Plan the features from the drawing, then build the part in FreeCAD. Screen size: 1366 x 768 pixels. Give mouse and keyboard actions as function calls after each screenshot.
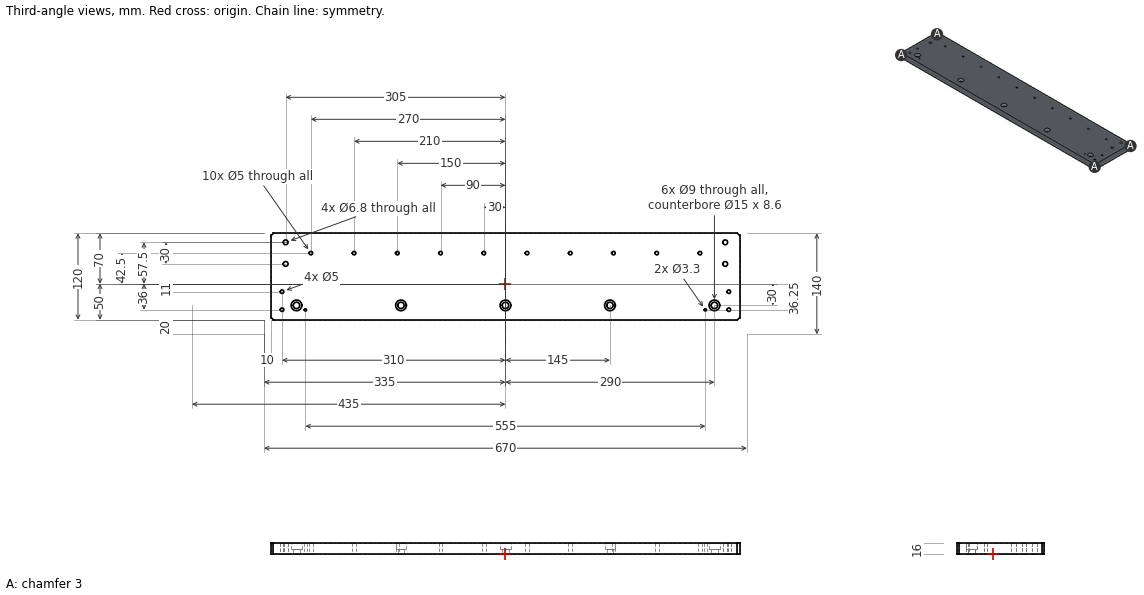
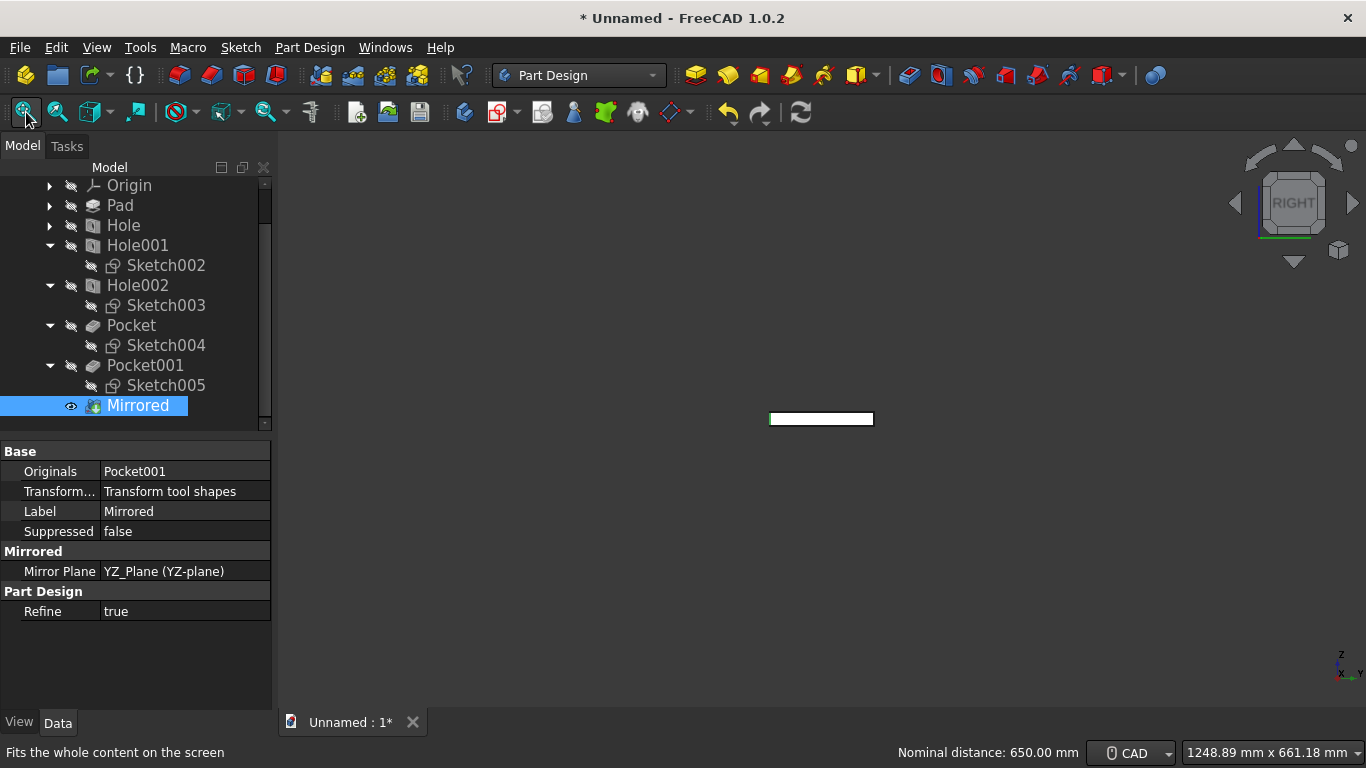
click(874, 418, ctrl)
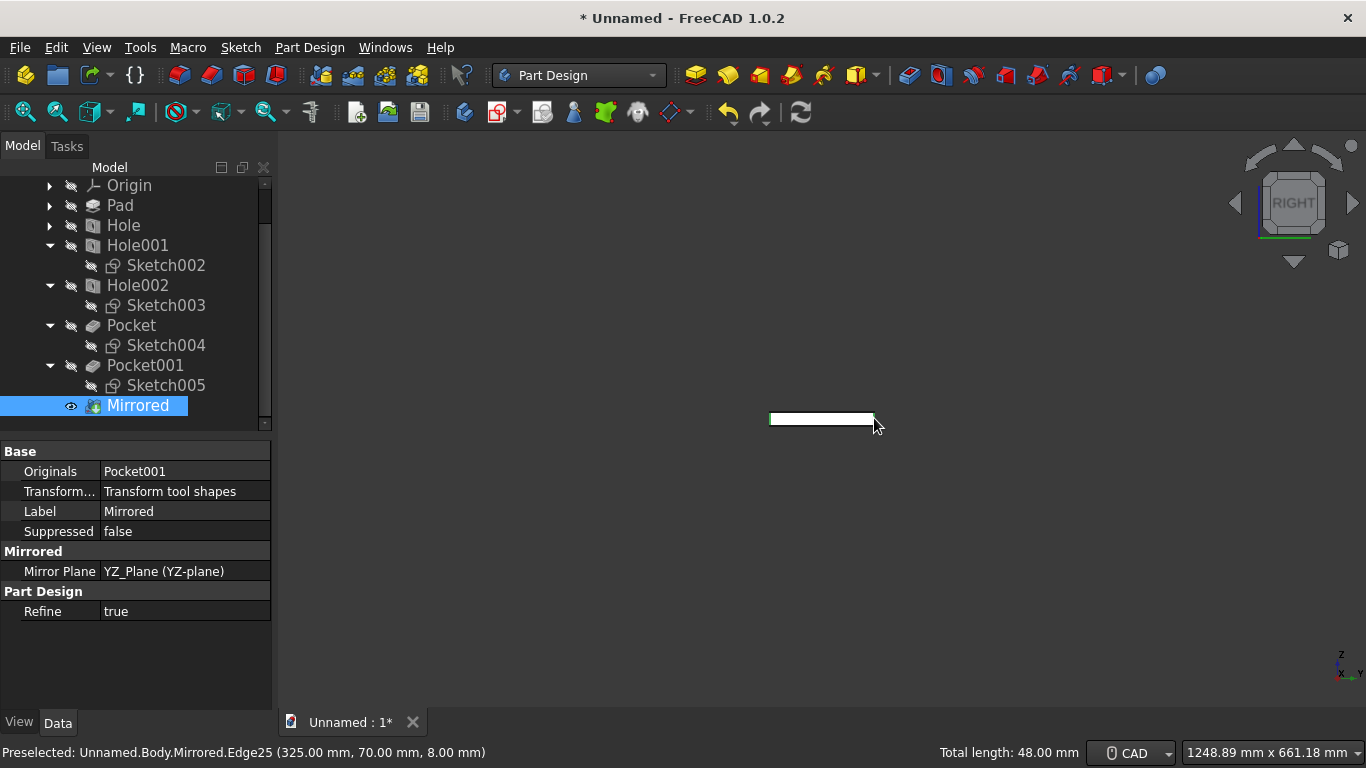
scroll(874, 418, up, 6)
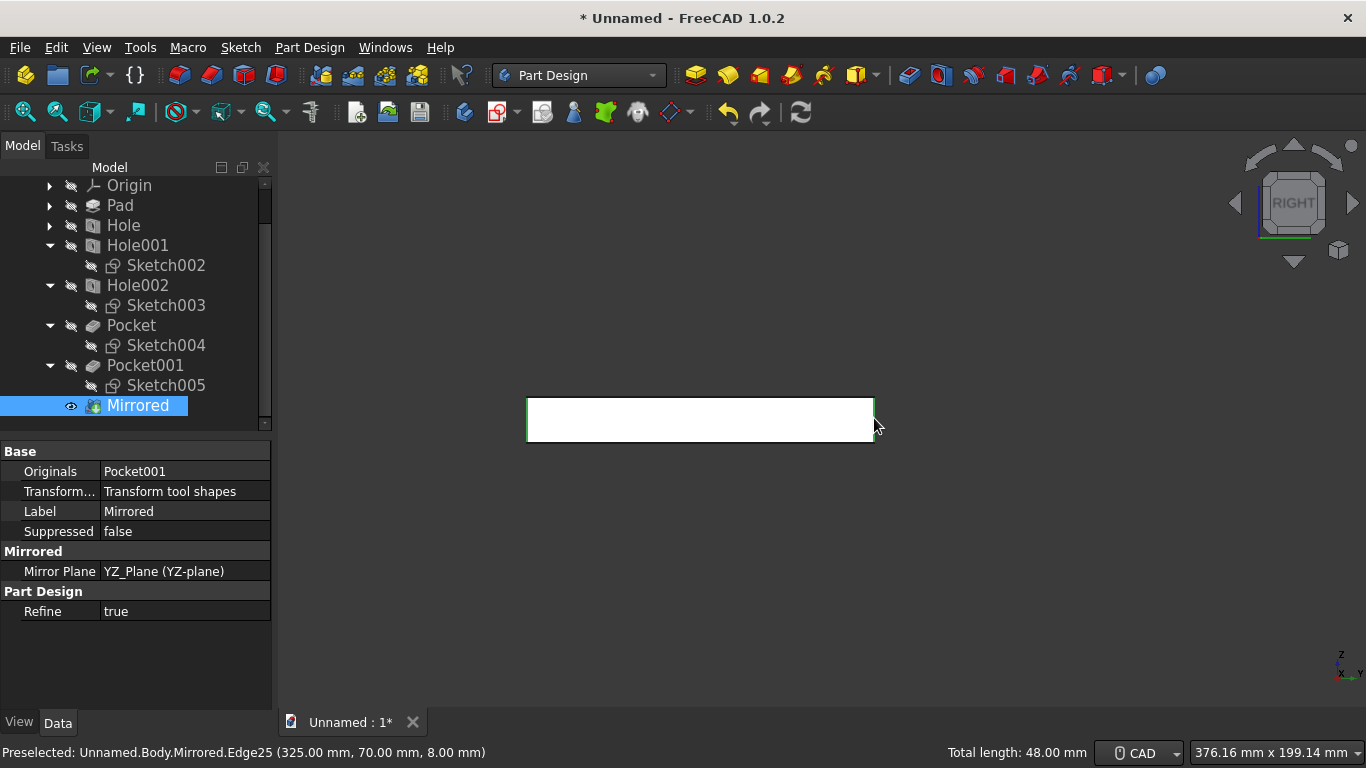
click(26, 112)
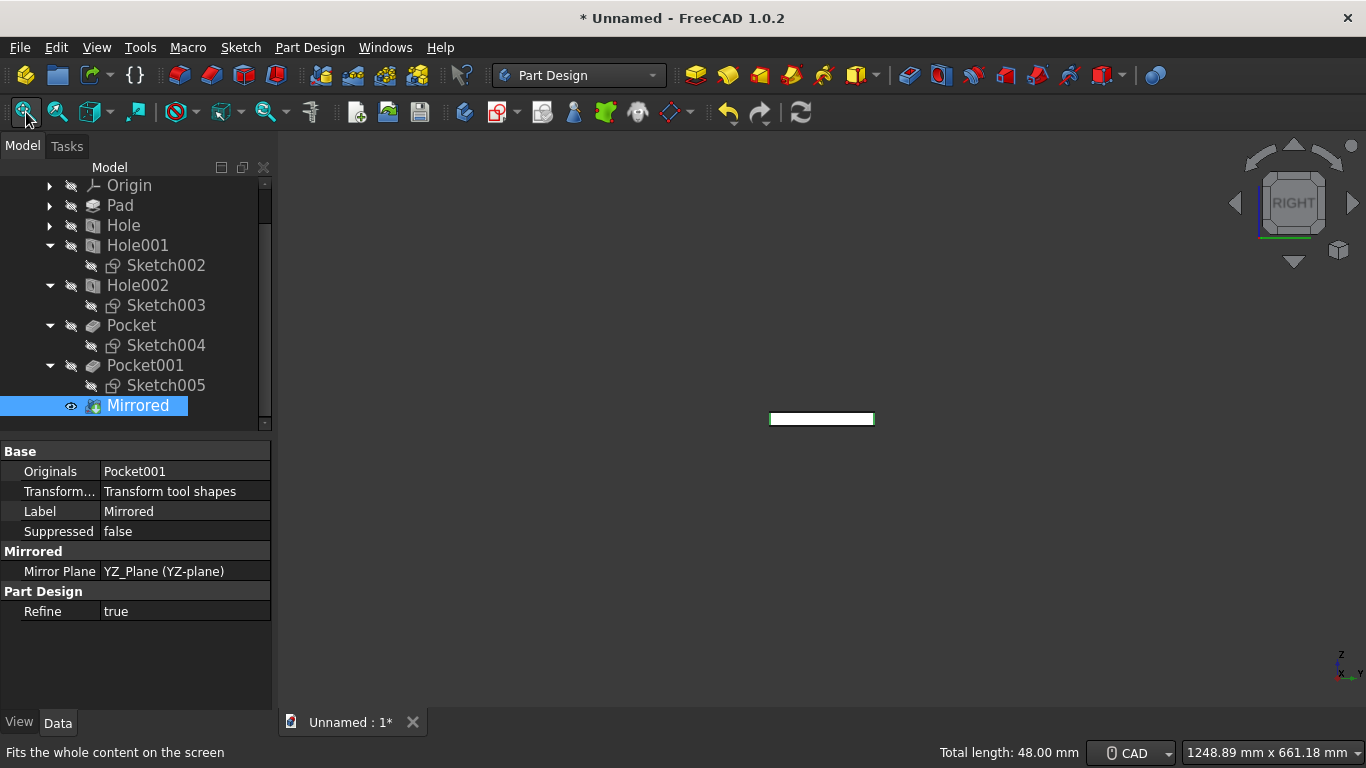
key(5)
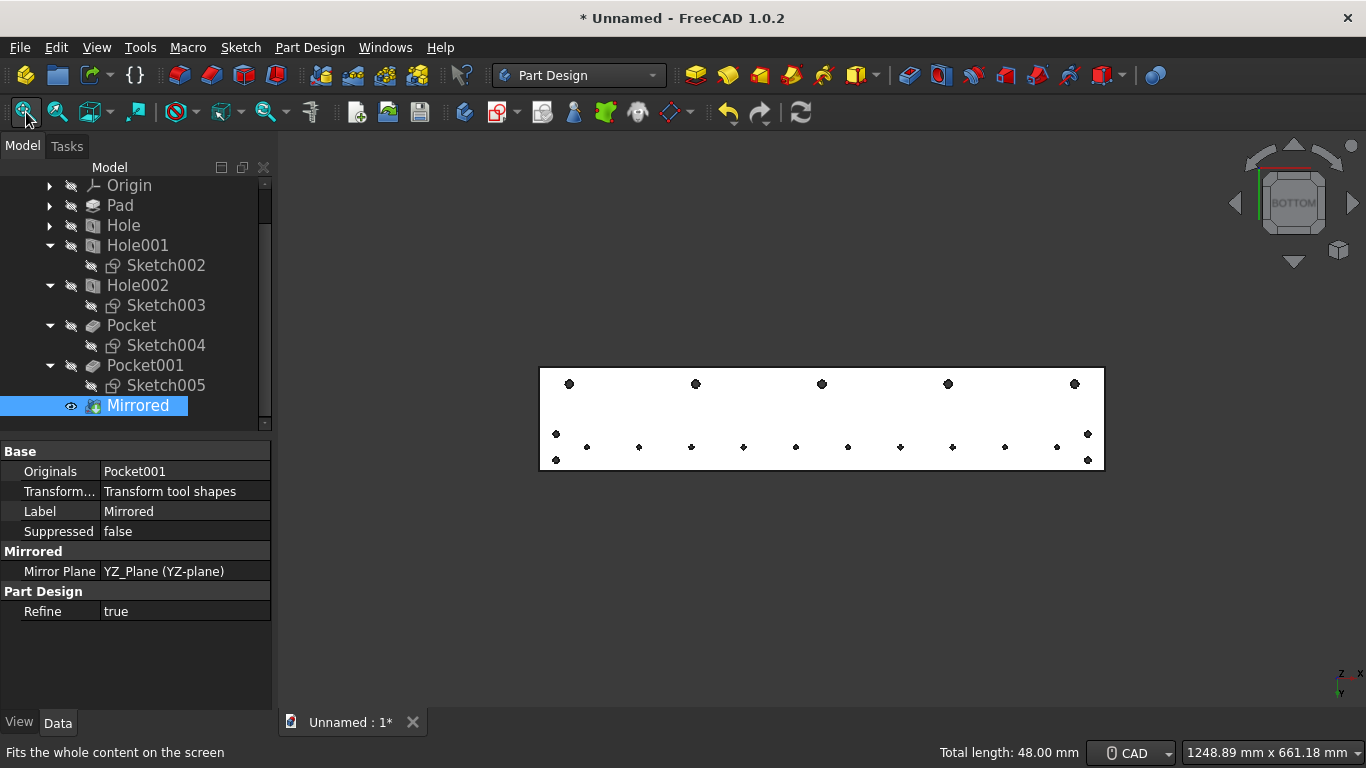
scroll(539, 470, up, 6)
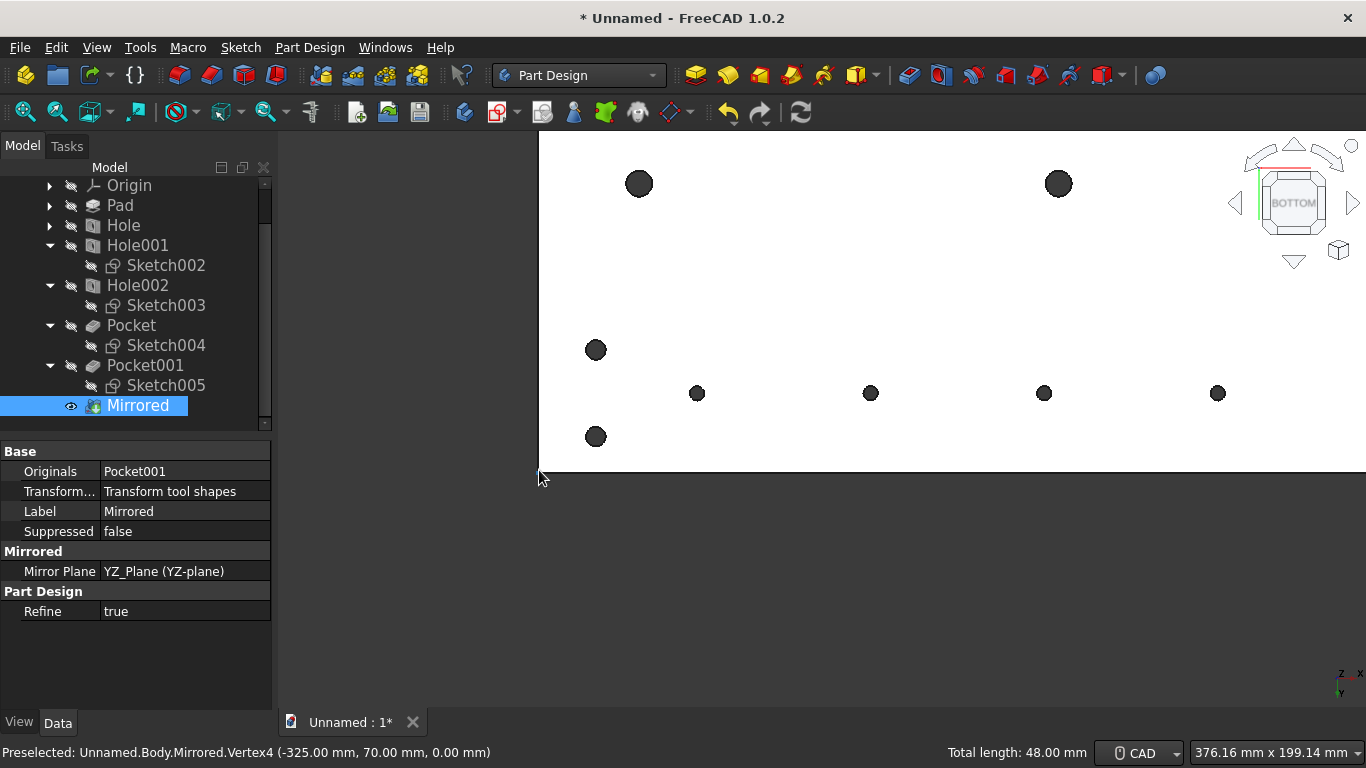
click(26, 112)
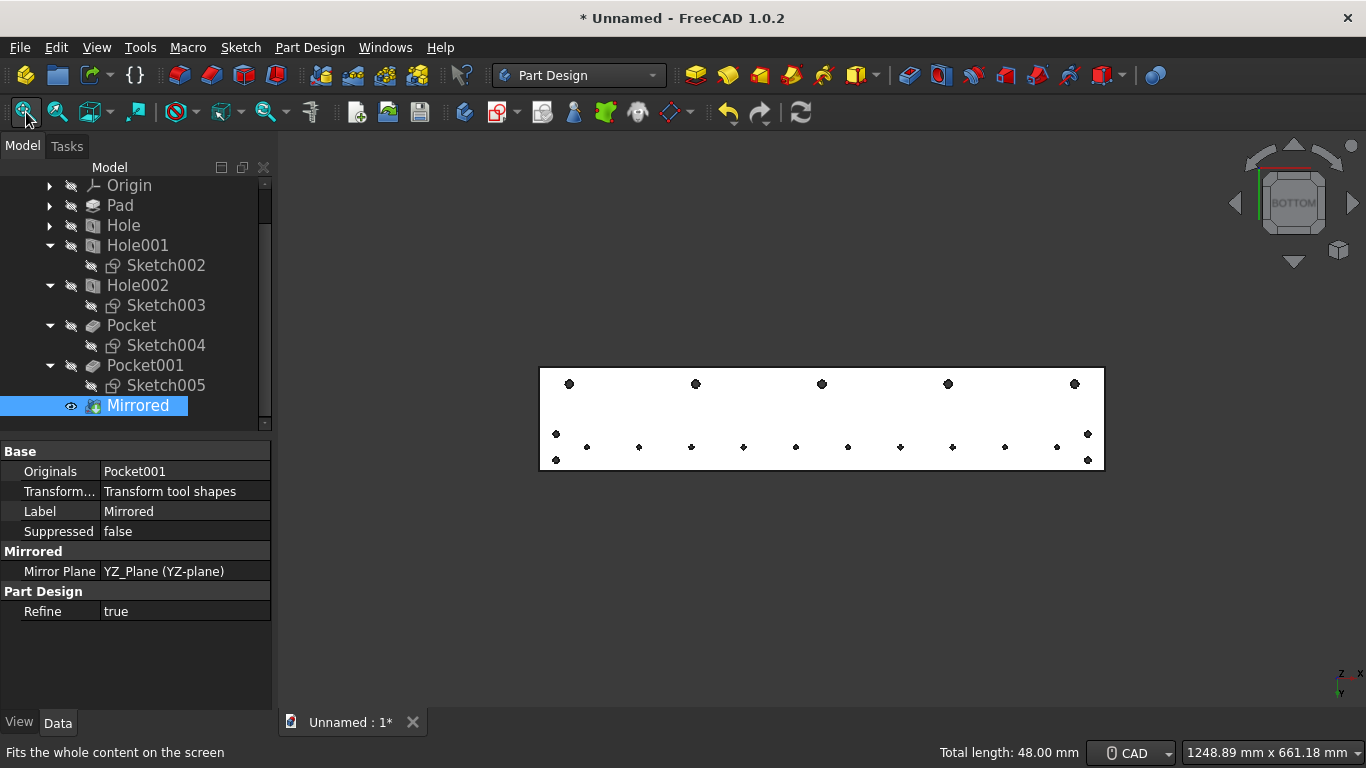
key(4)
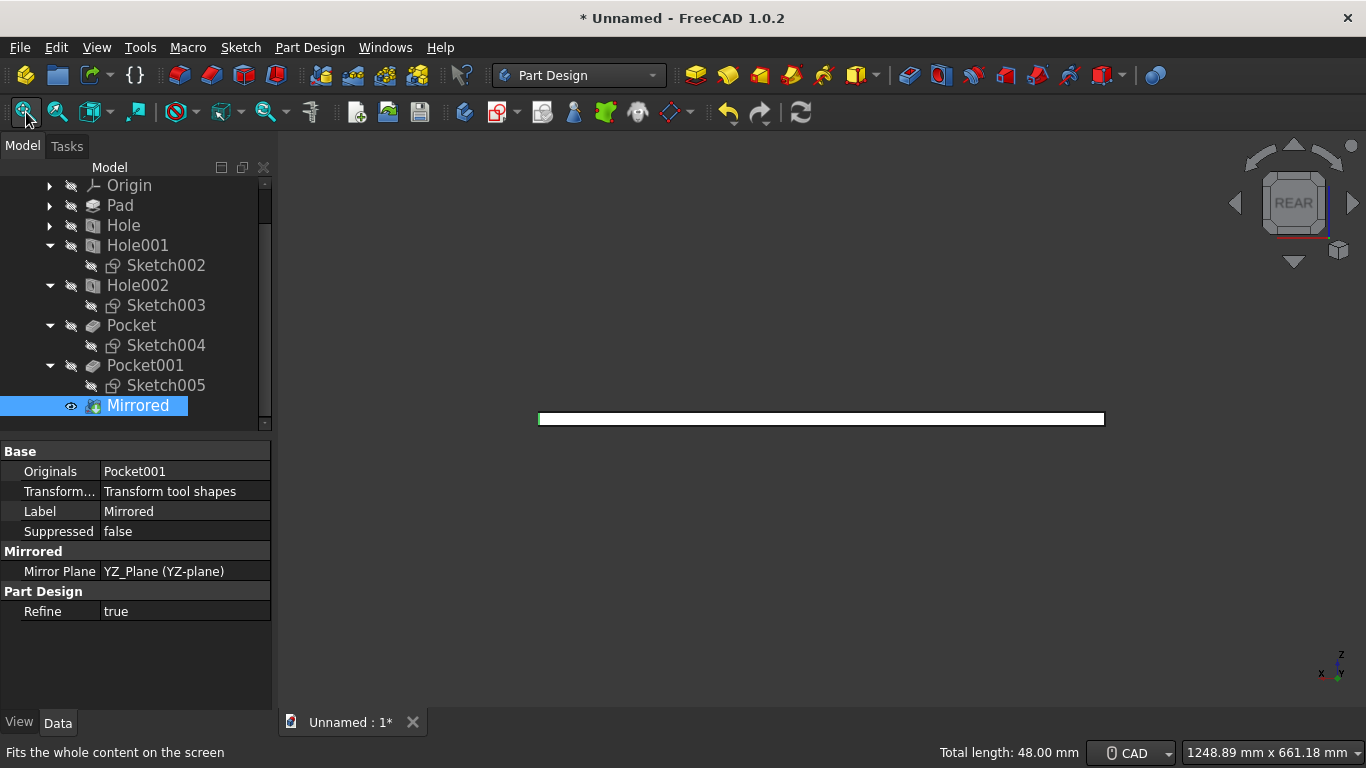
click(1105, 418, ctrl)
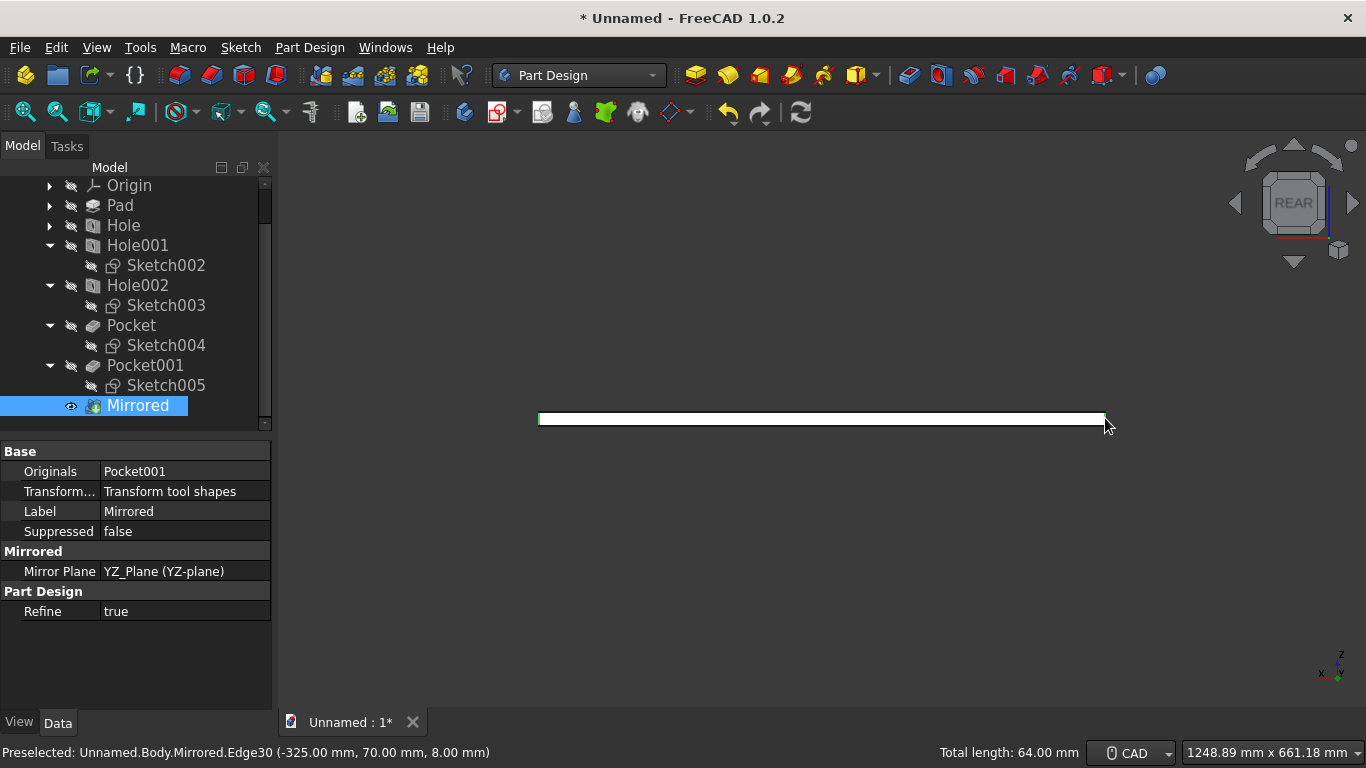
click(212, 76)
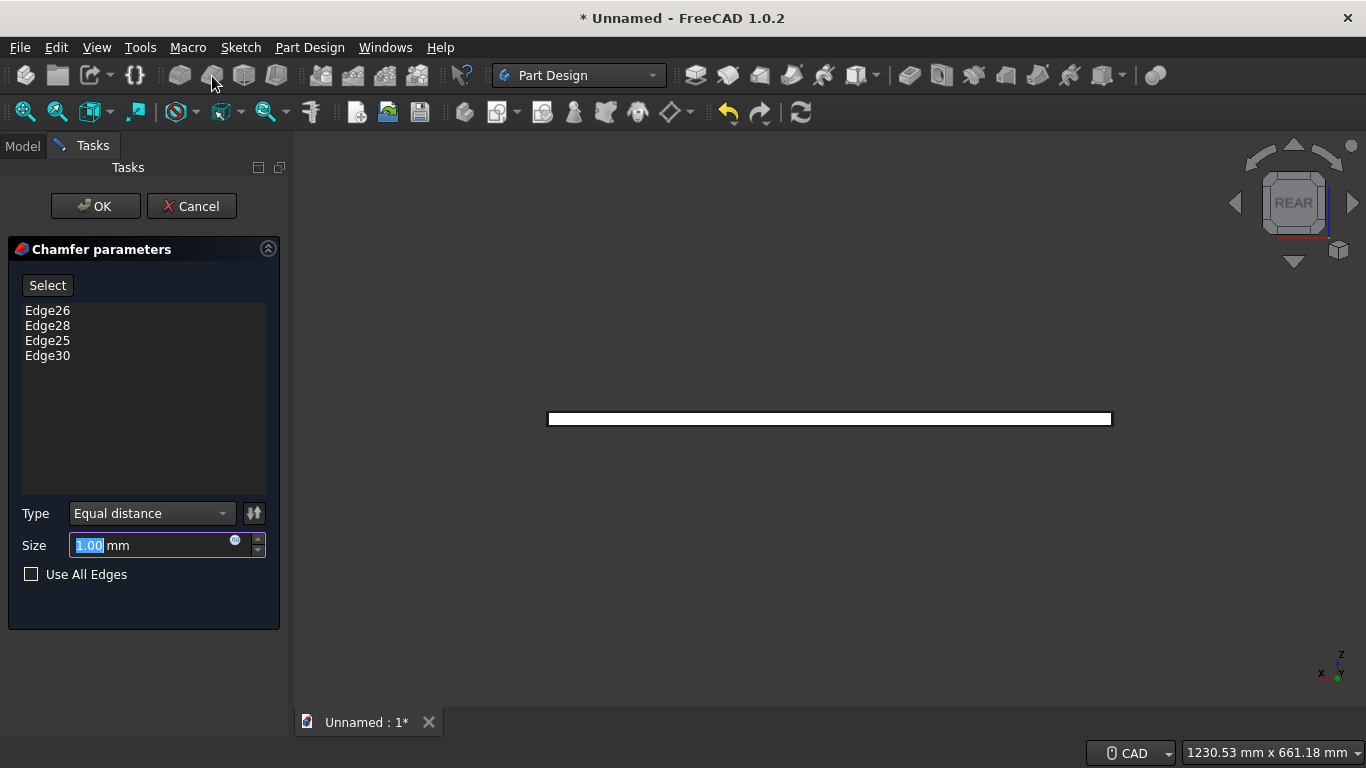
text(3)
key(Tab)